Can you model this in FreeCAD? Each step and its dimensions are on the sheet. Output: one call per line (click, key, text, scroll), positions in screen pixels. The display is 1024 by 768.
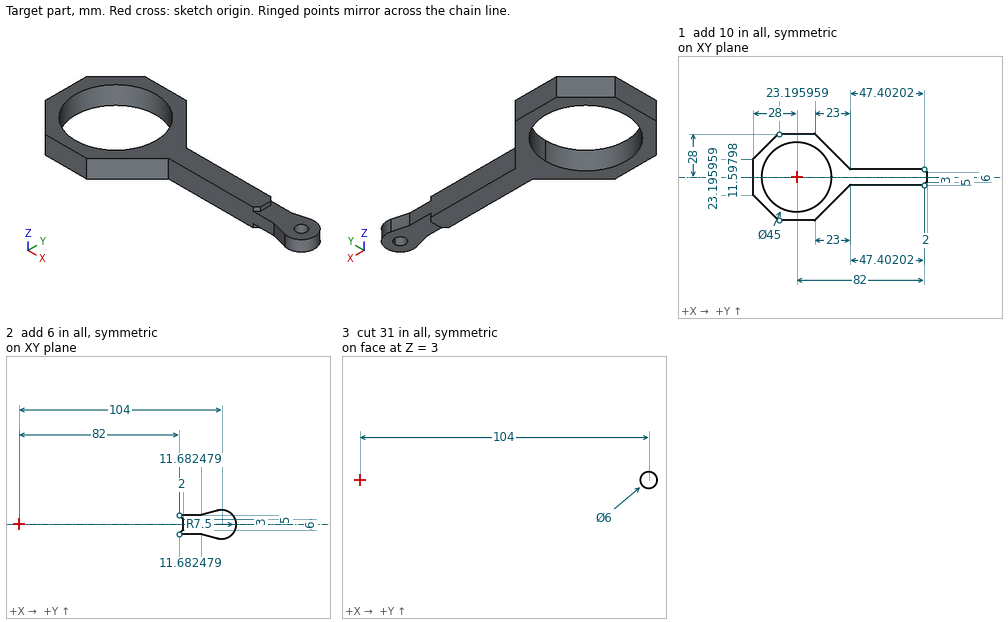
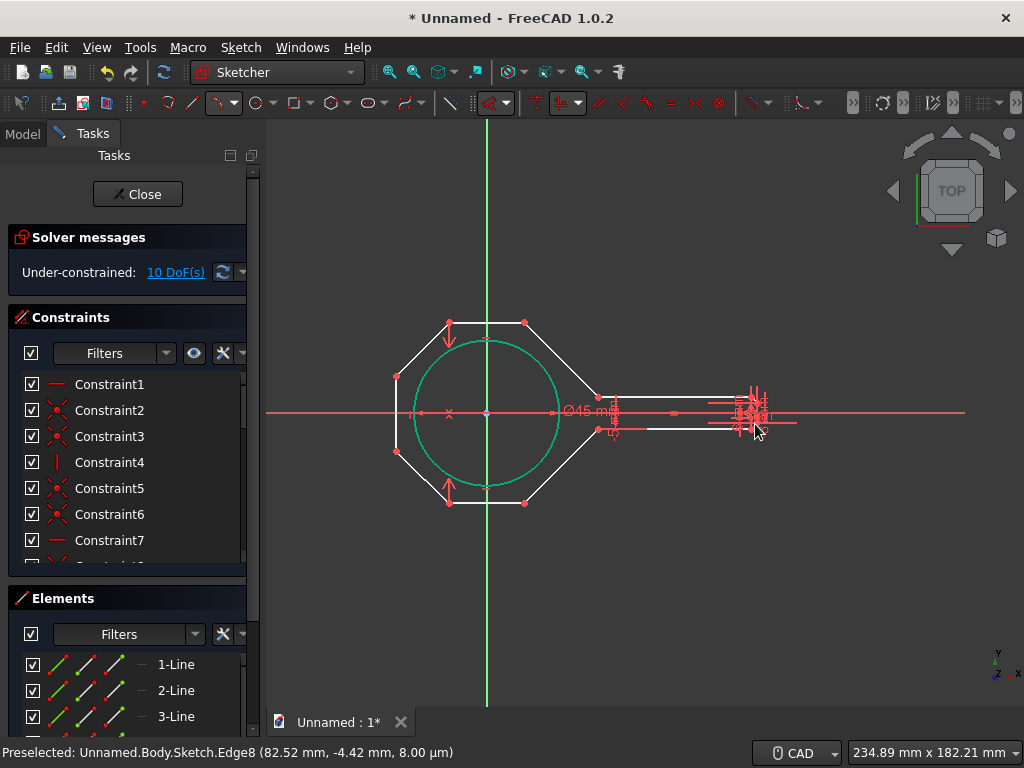
click(524, 323)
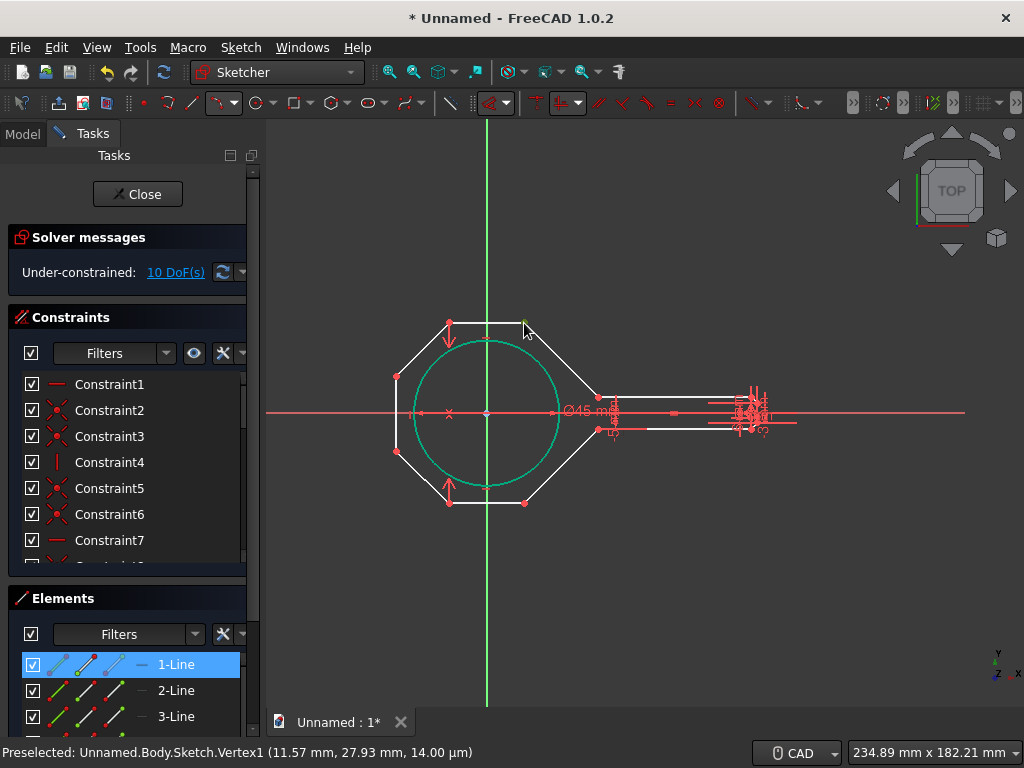
click(508, 104)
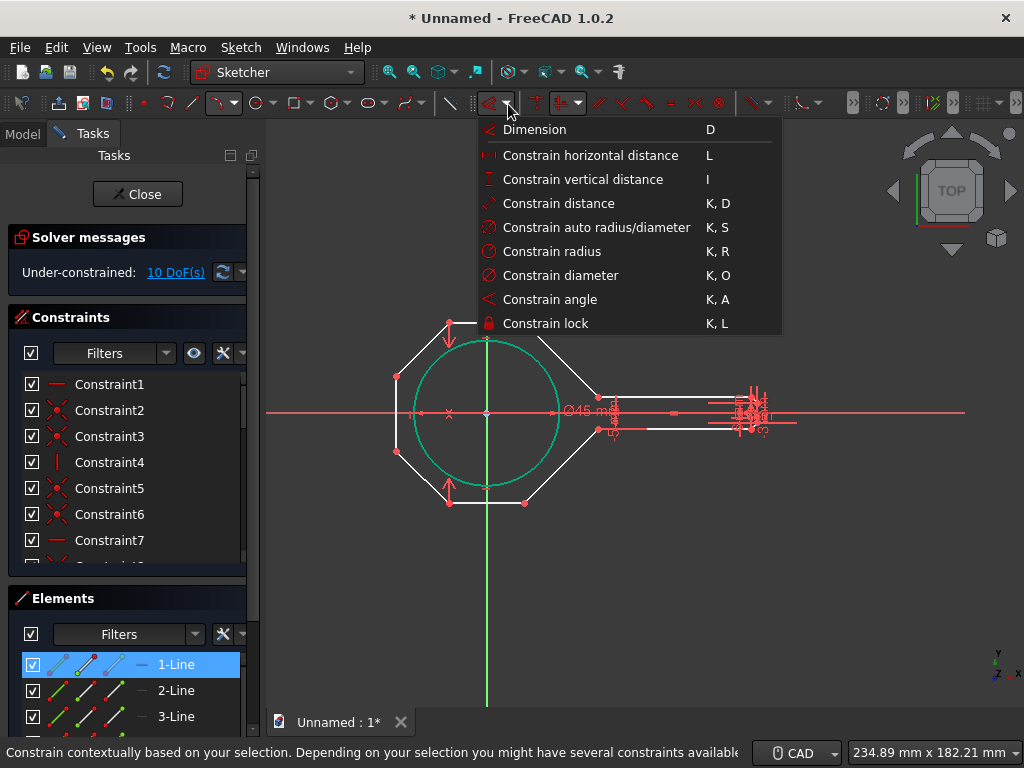
click(630, 179)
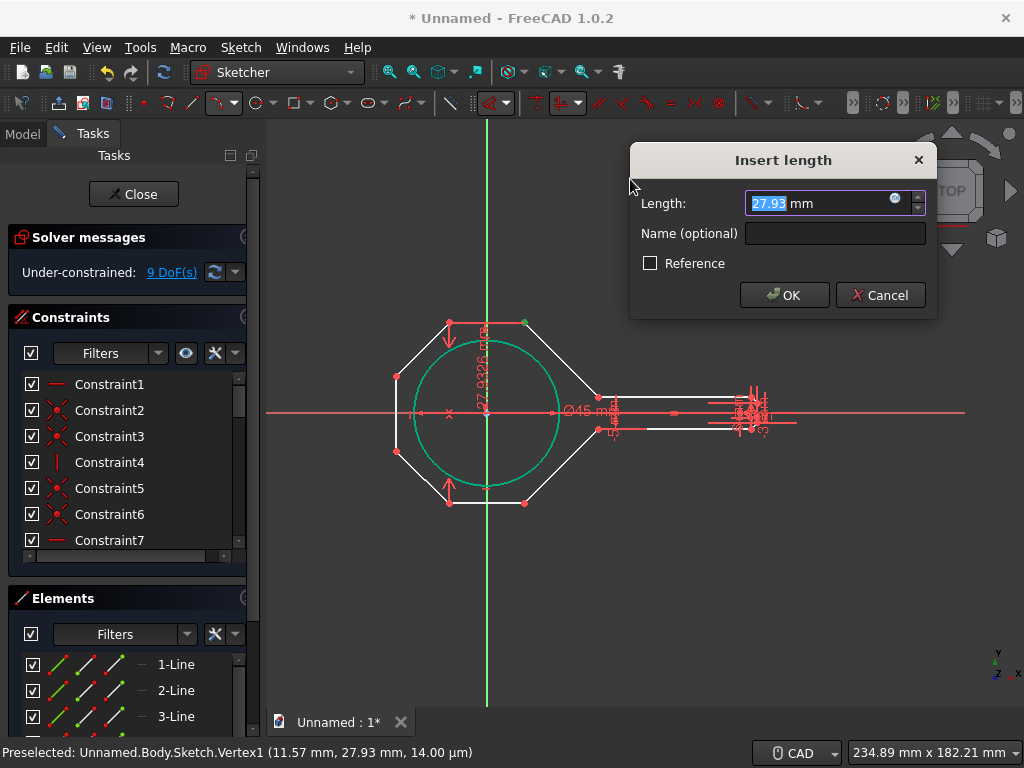
text(28)
key(Return)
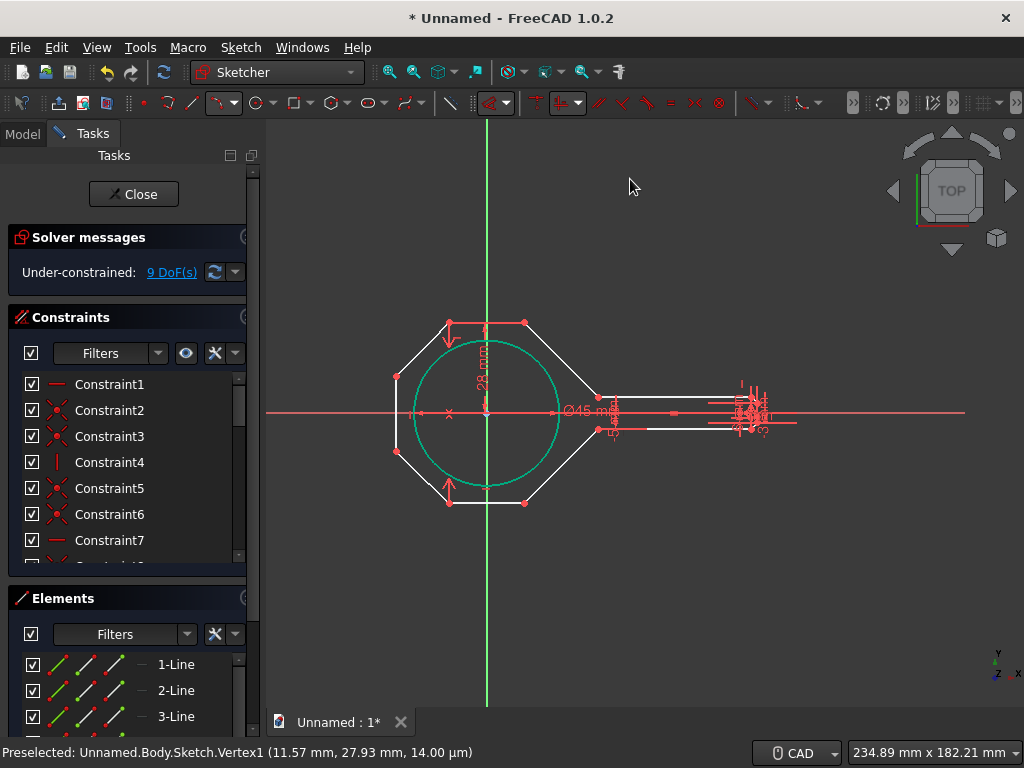
click(396, 377)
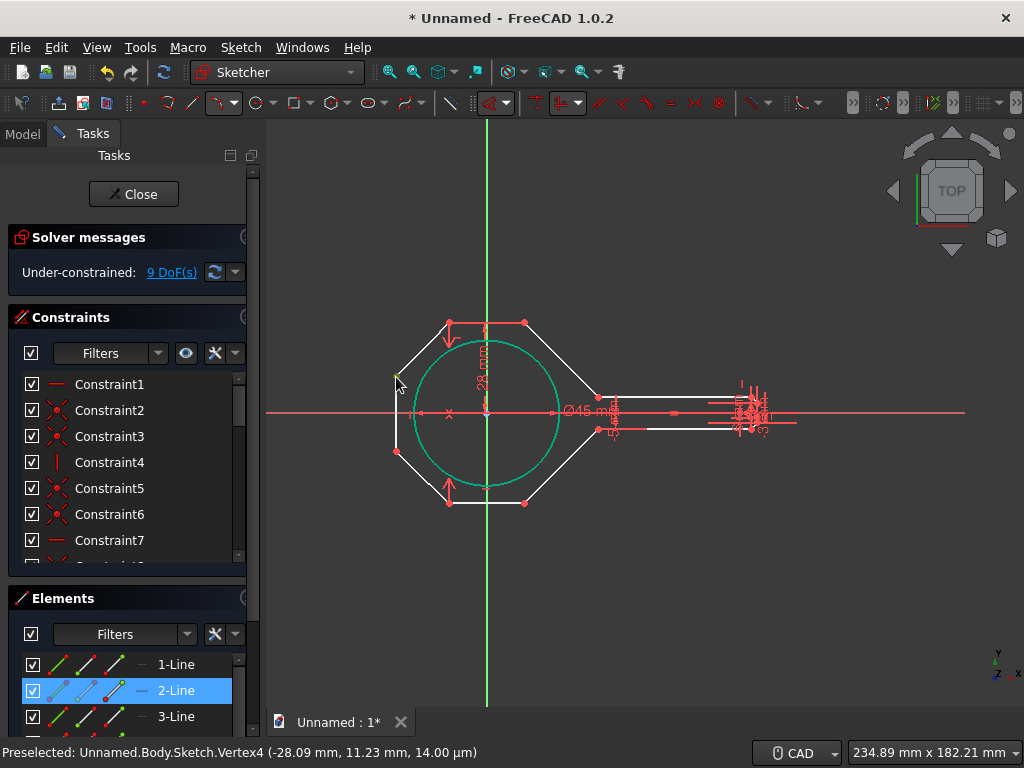
key(l)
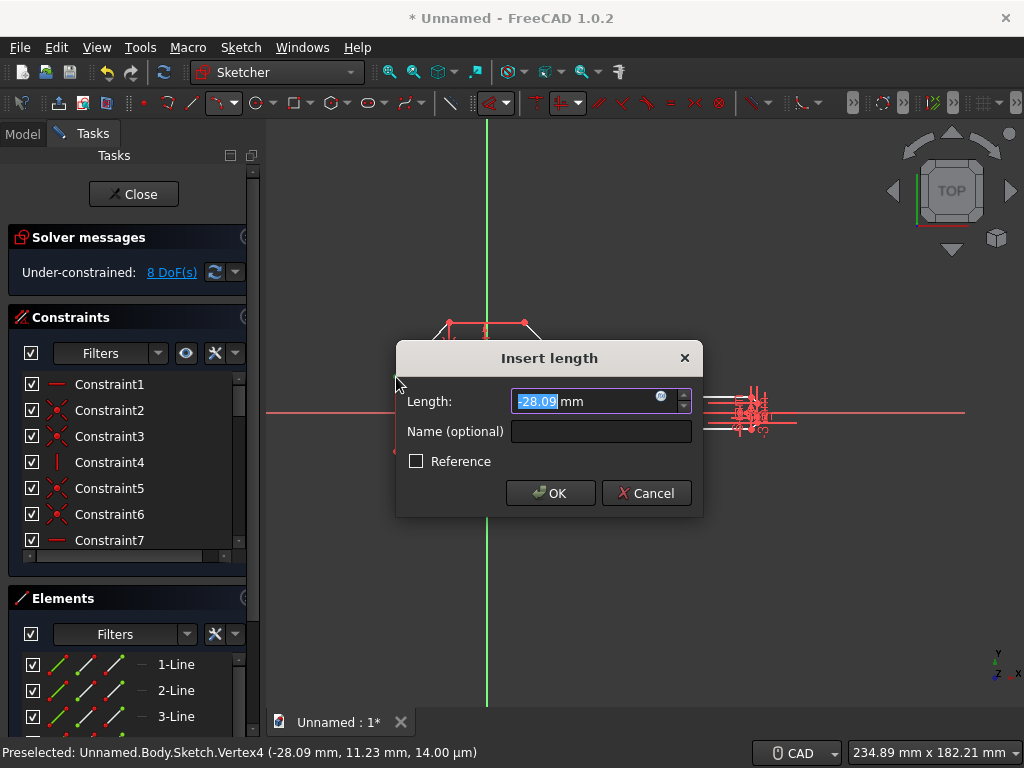
text(-28)
key(Return)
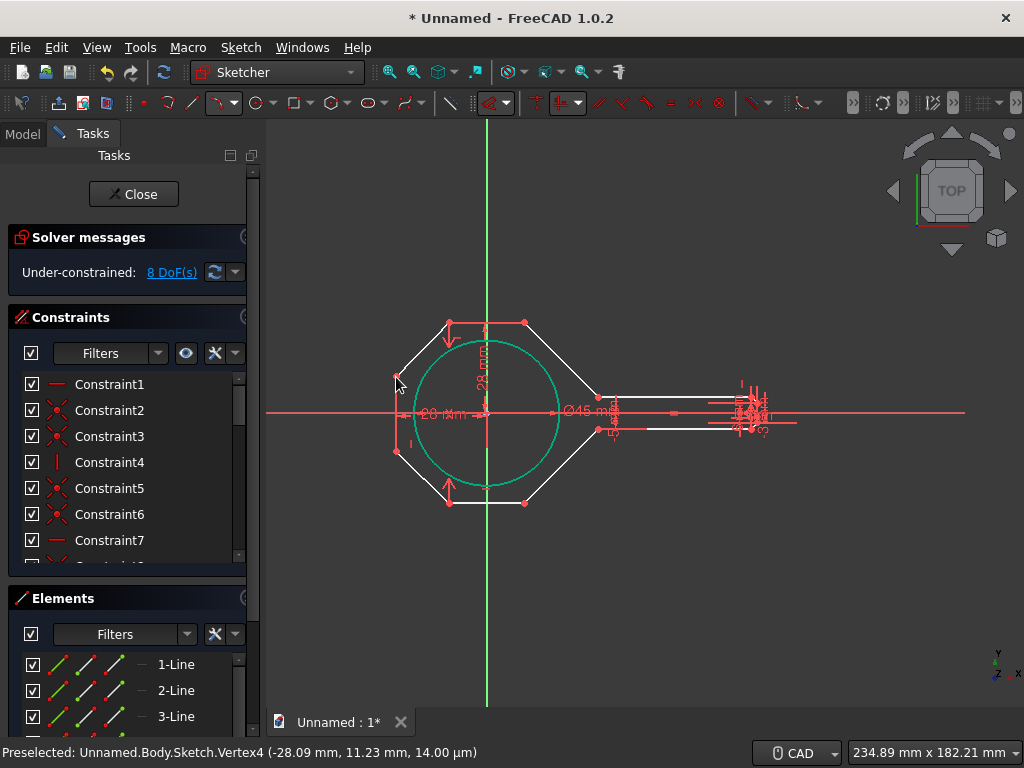
scroll(751, 429, up, 2)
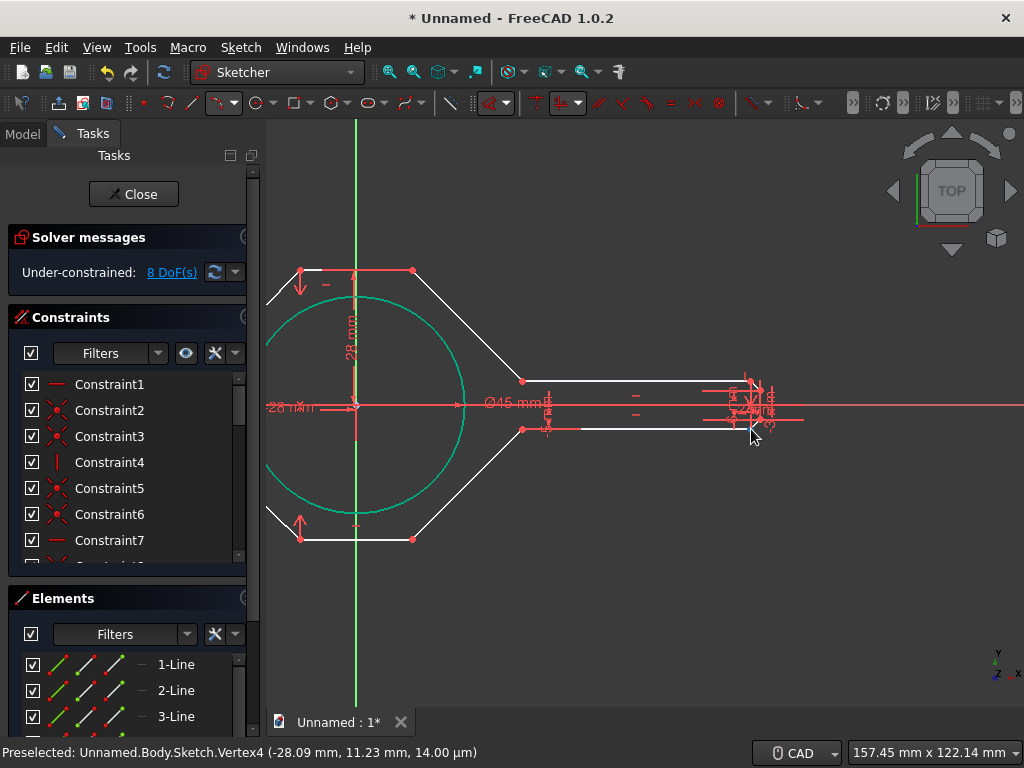
click(751, 429)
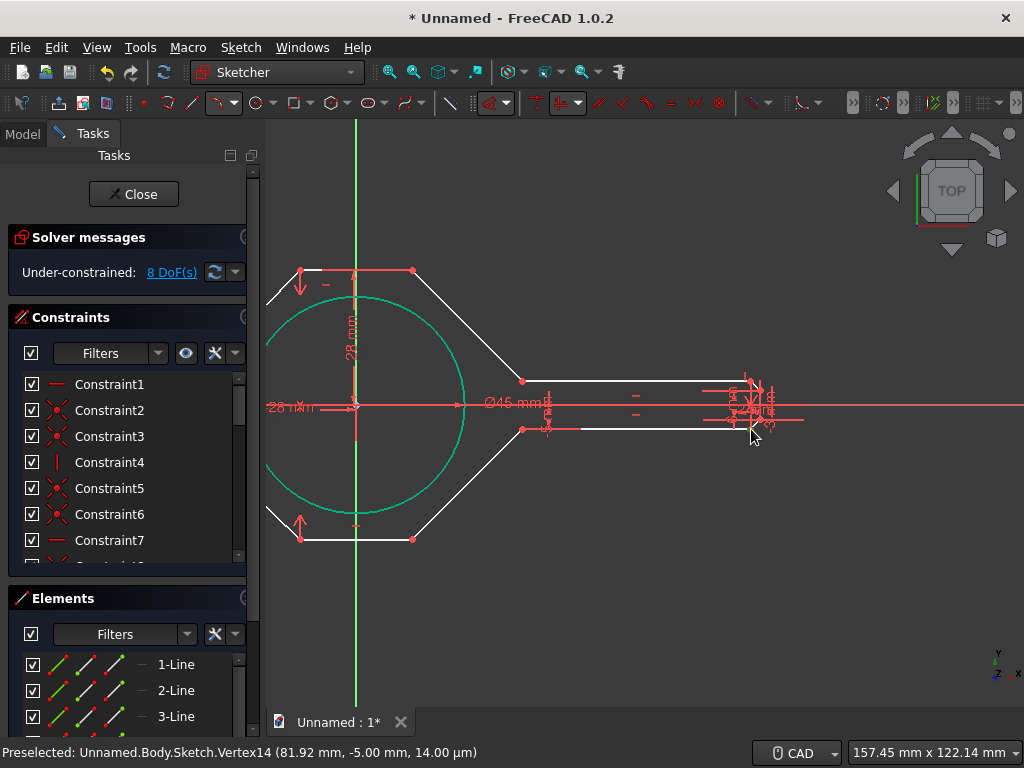
click(508, 104)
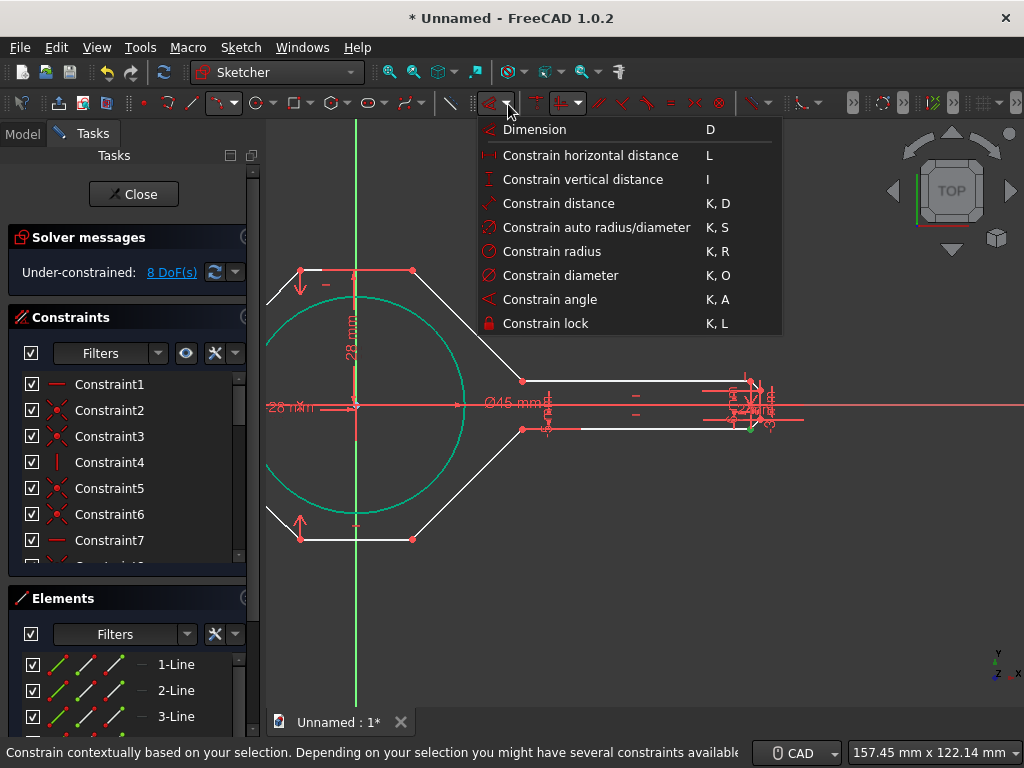
click(630, 155)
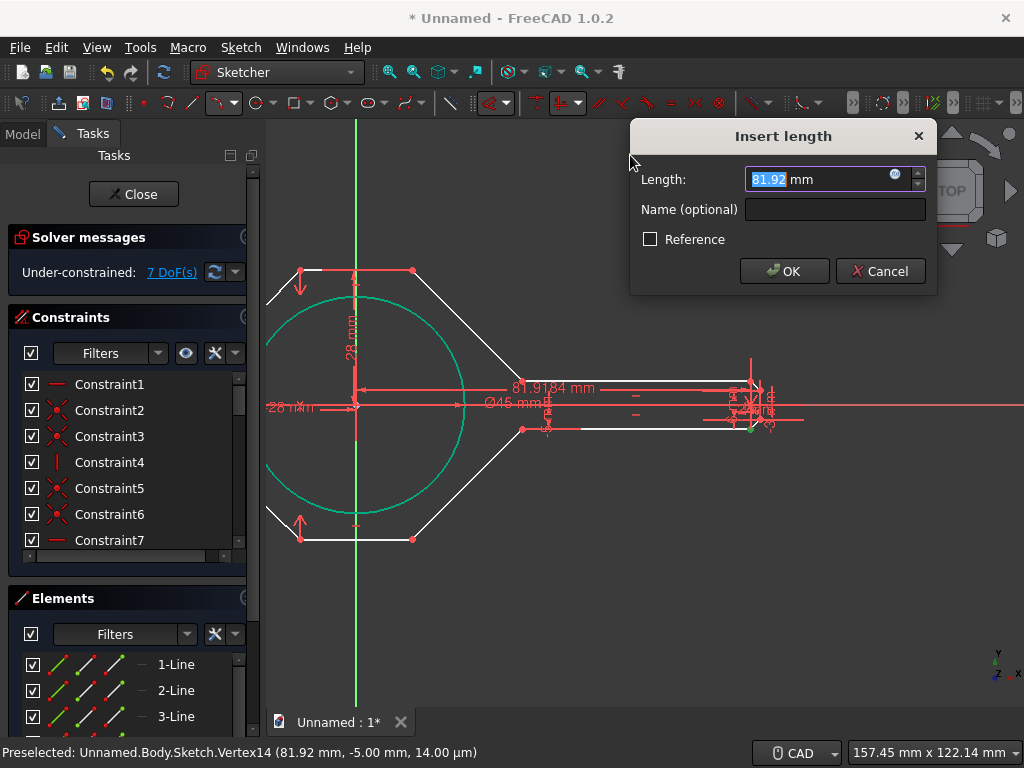
text(82)
key(Return)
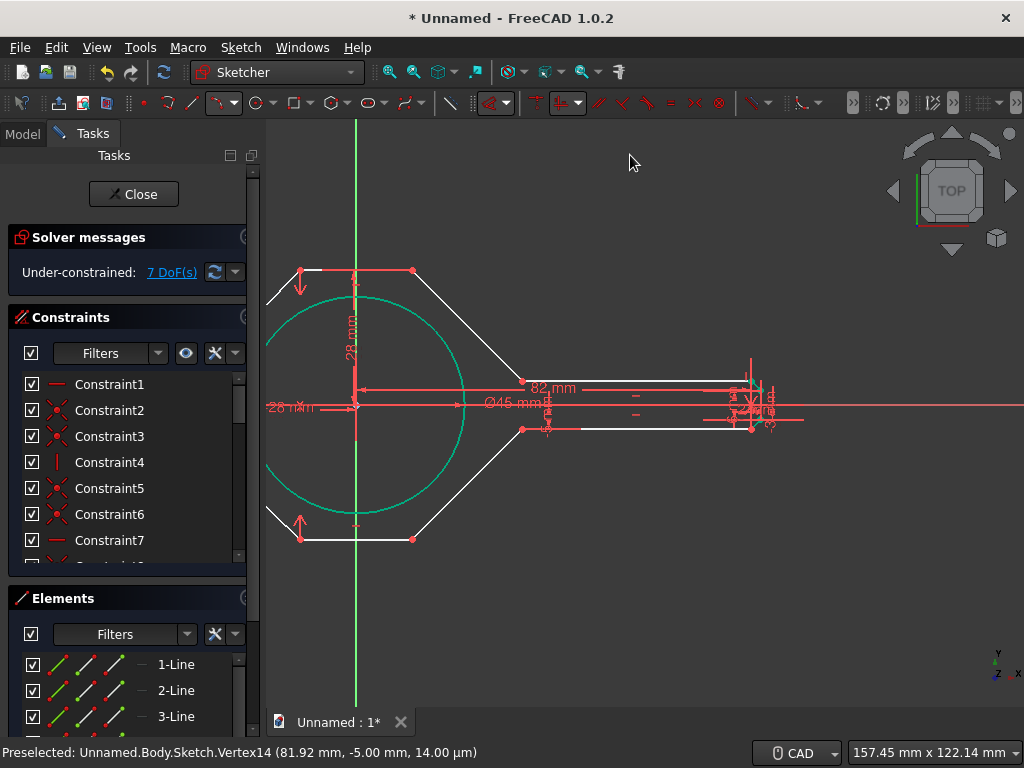
click(445, 507)